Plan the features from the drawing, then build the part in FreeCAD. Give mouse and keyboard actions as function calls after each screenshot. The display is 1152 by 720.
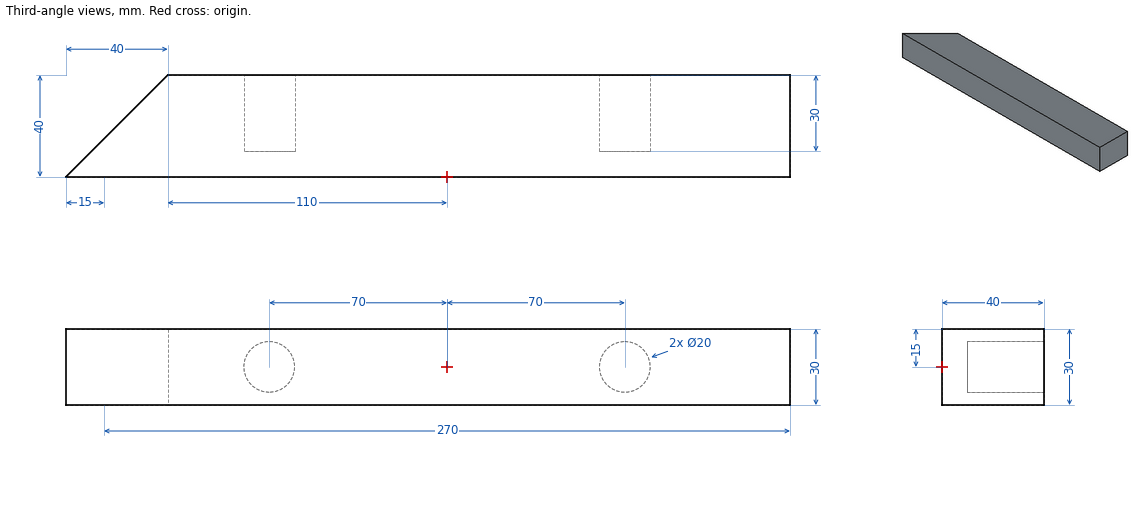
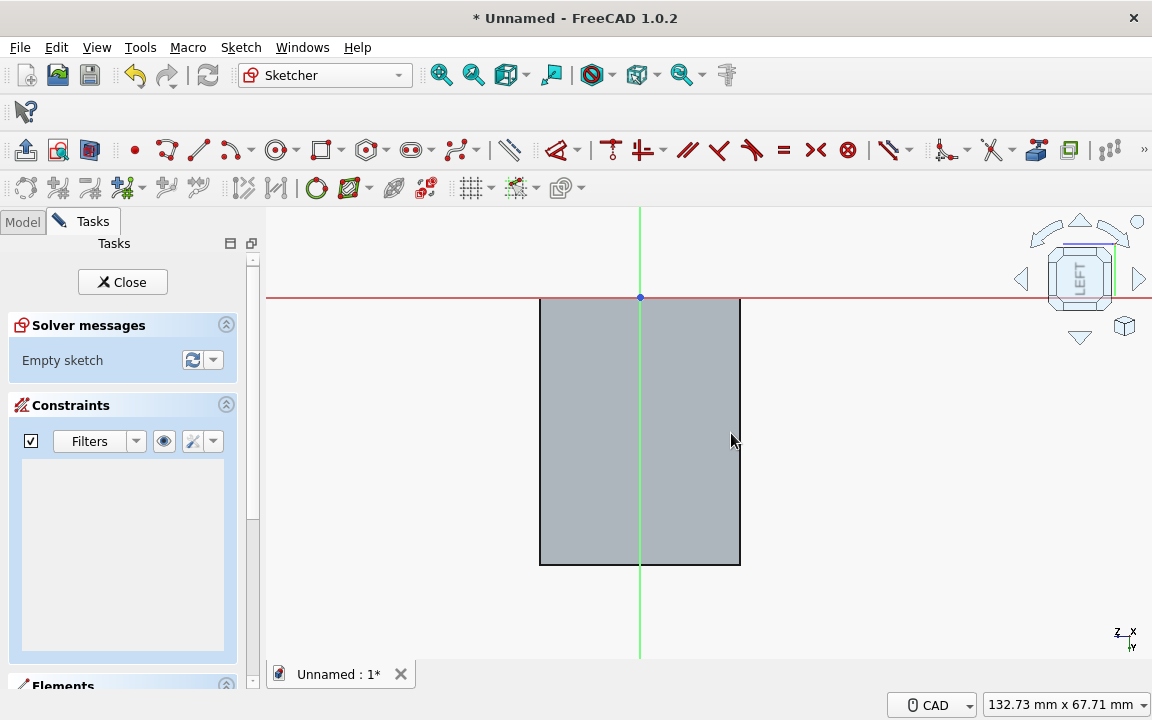
key(g)
key(r)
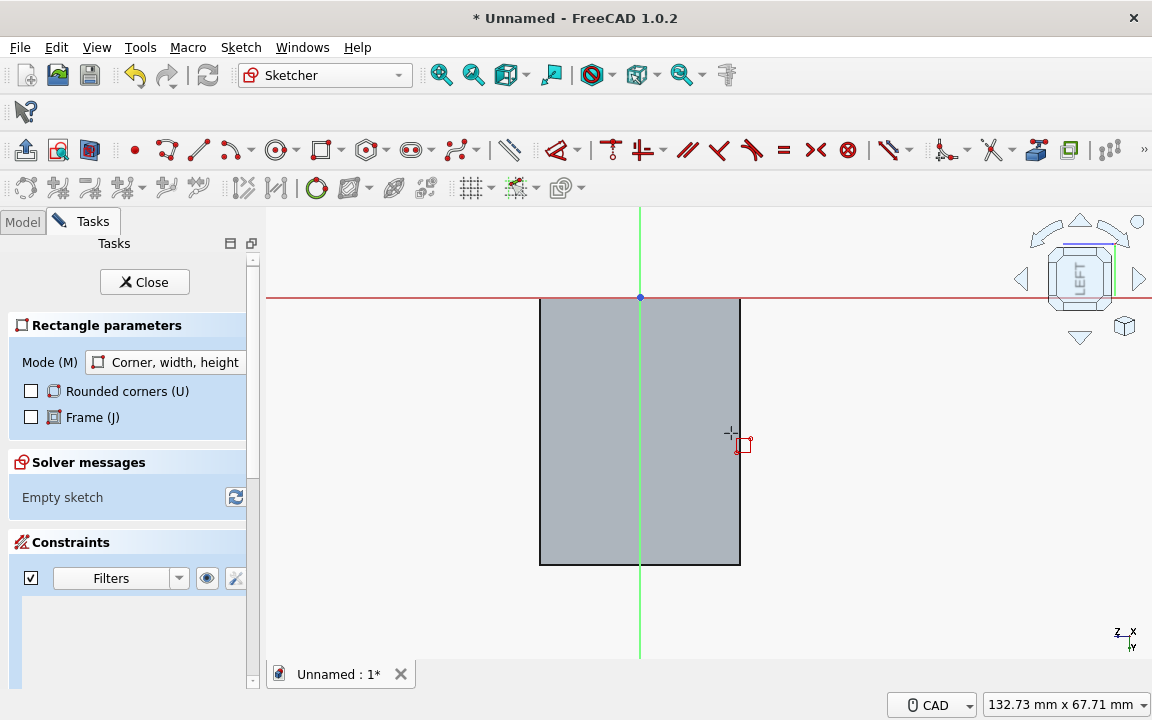
click(540, 298)
move(740, 565)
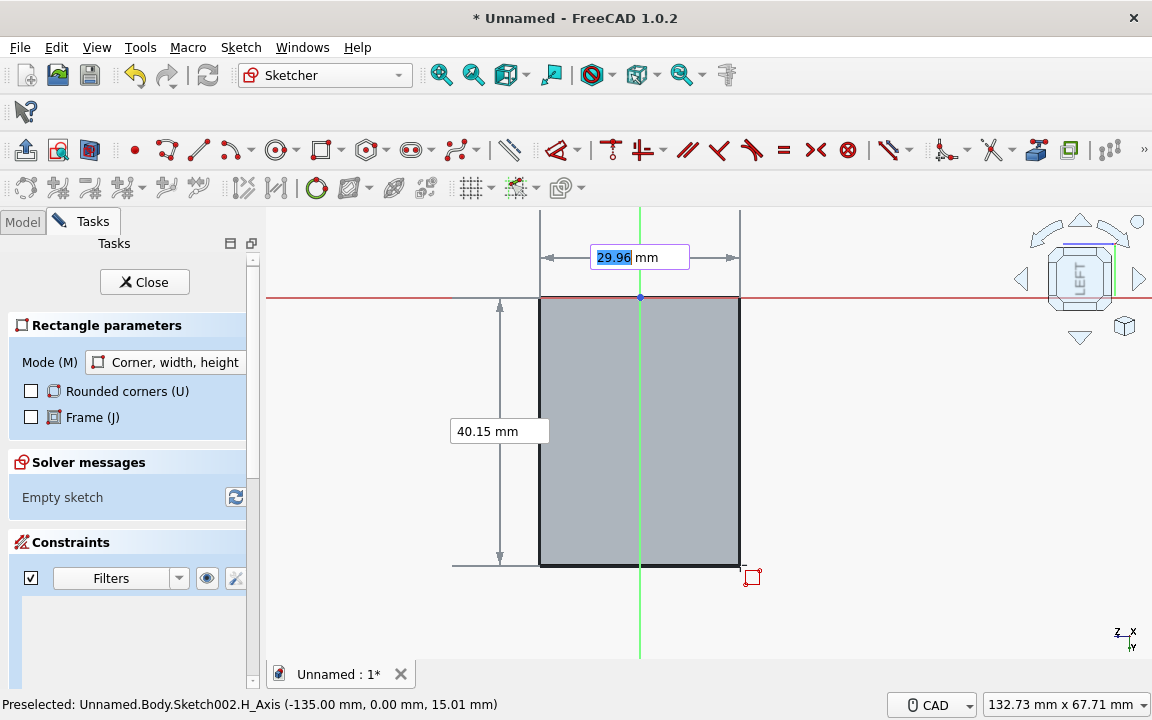
text(30)
key(Tab)
text(40)
key(Return)
key(Escape)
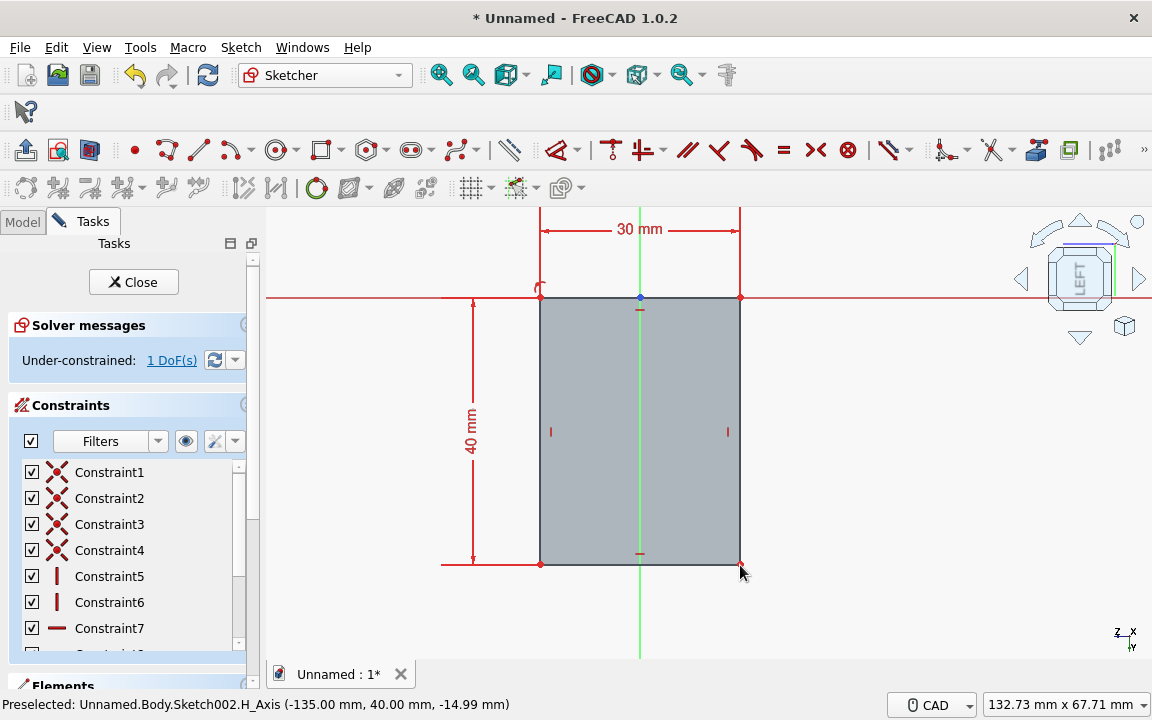
key(d)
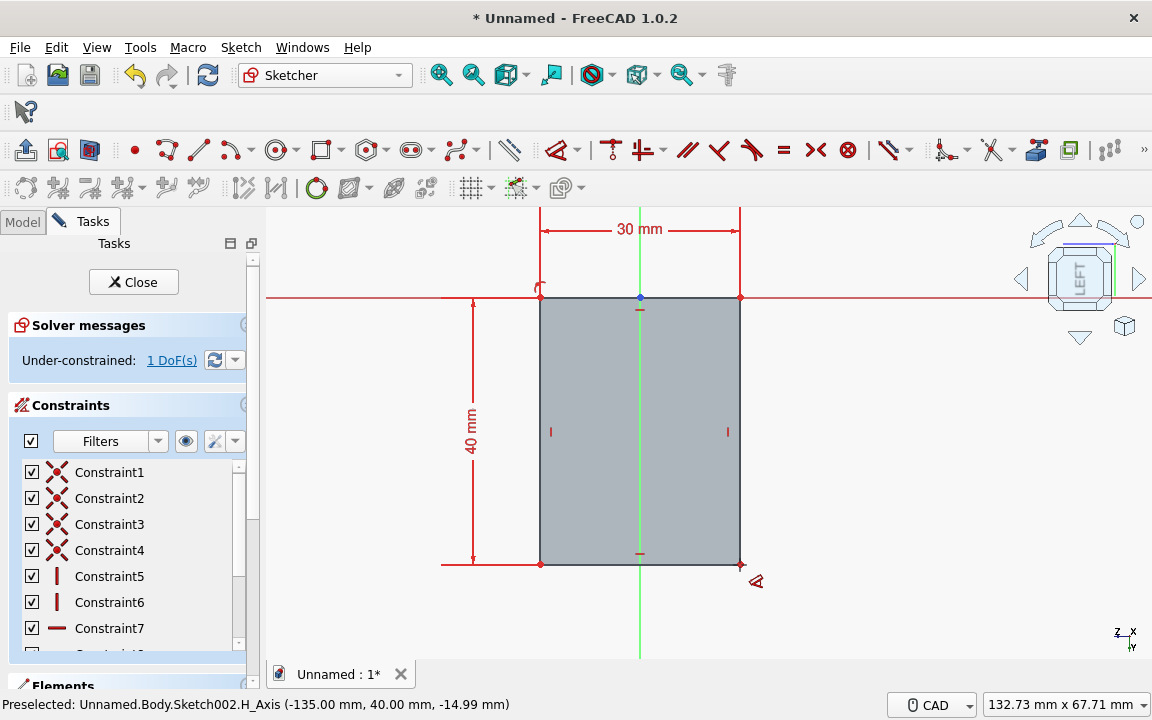
click(540, 298)
click(590, 264)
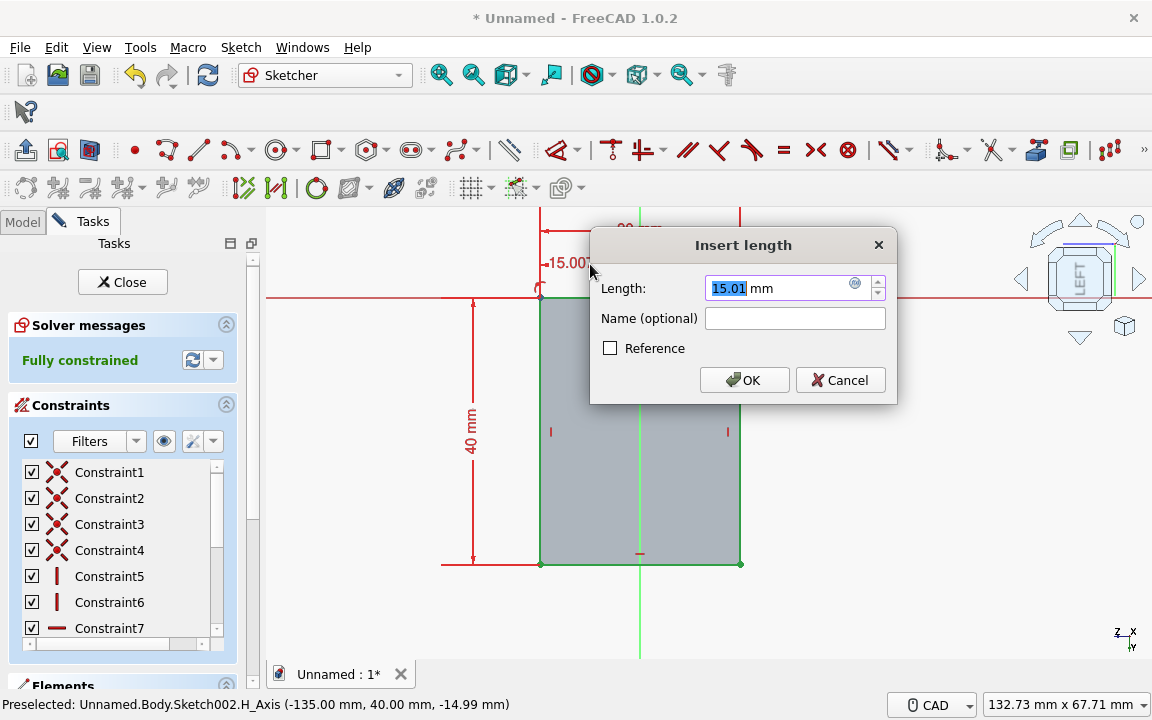
text(15)
key(Return)
key(Escape)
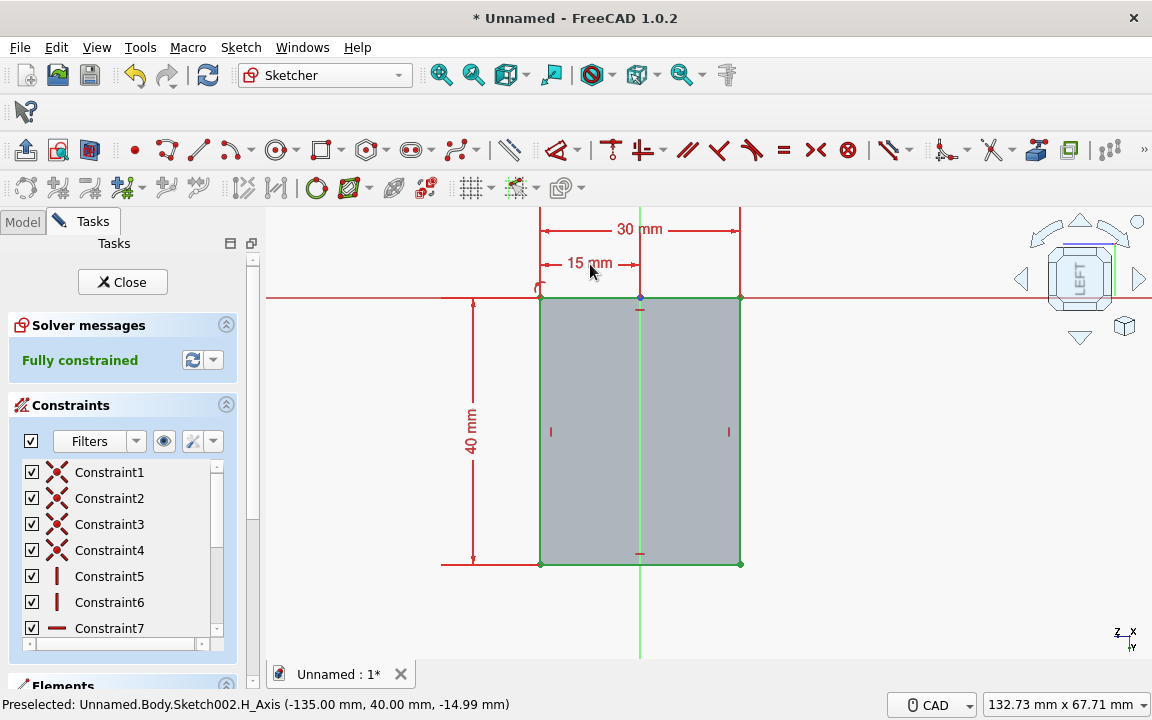
click(123, 282)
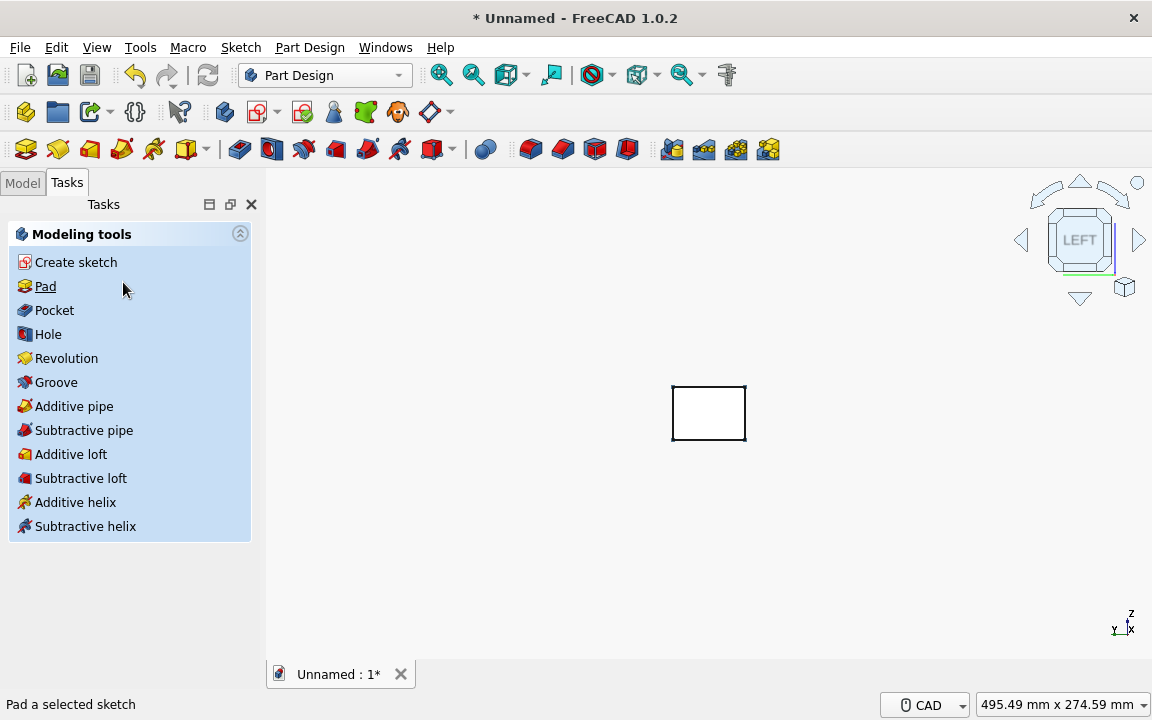
click(26, 150)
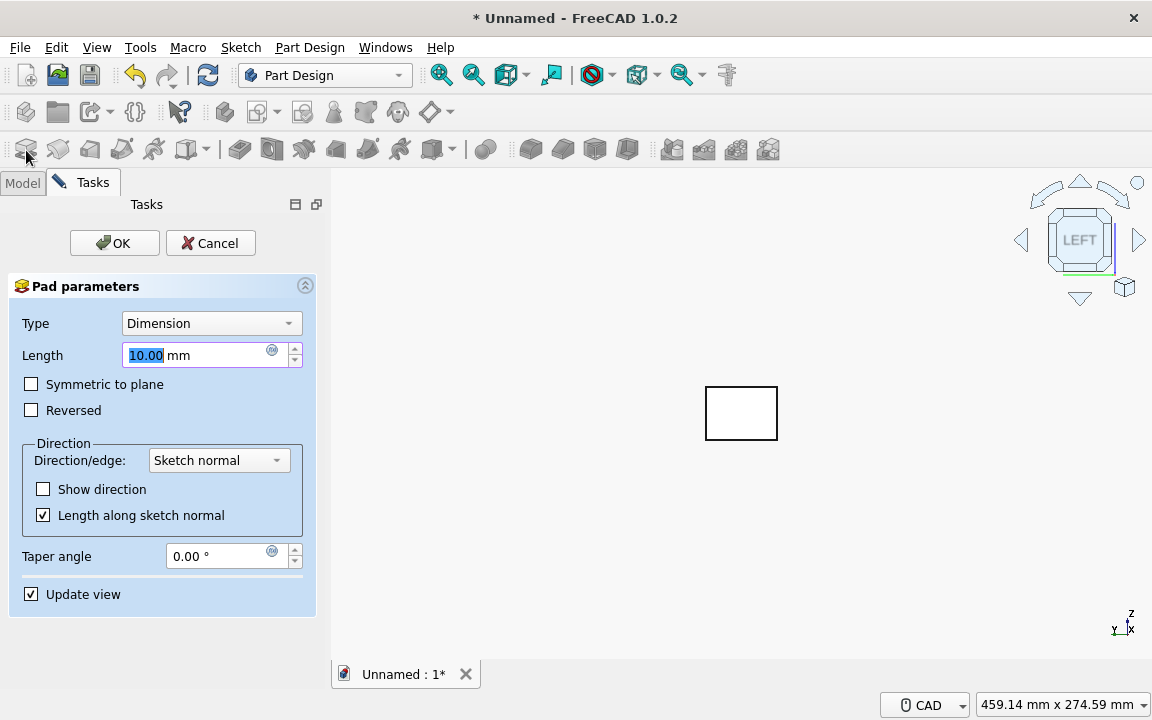
text(15)
key(Tab)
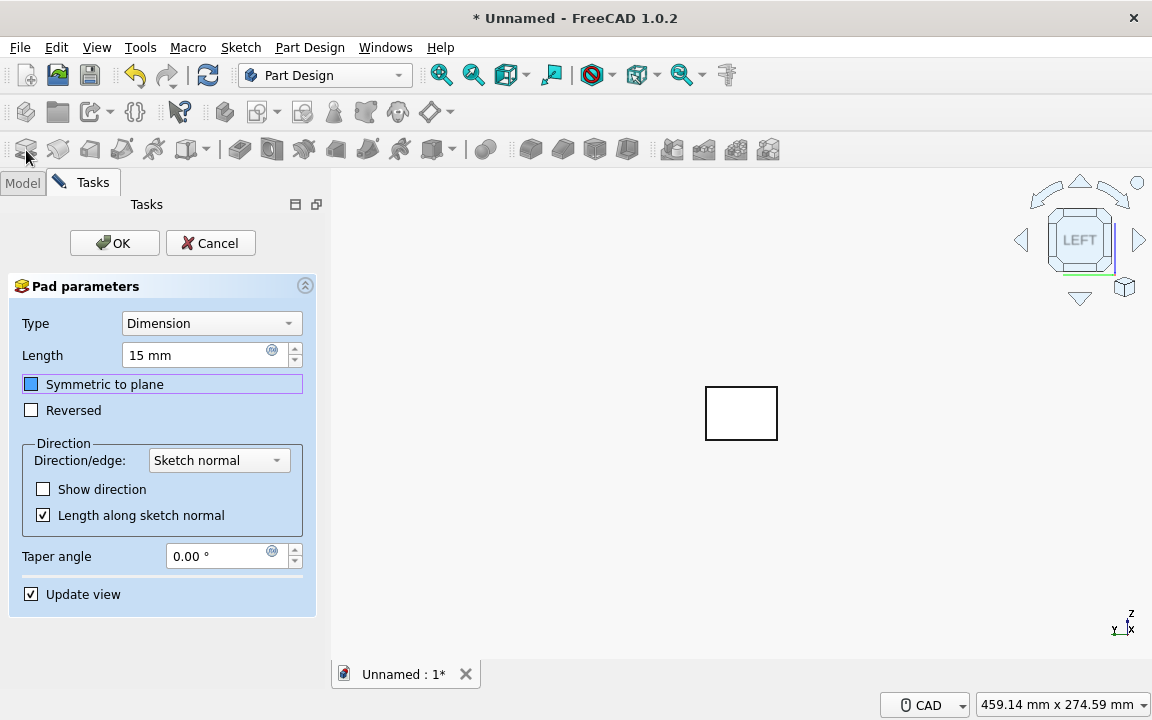
click(115, 243)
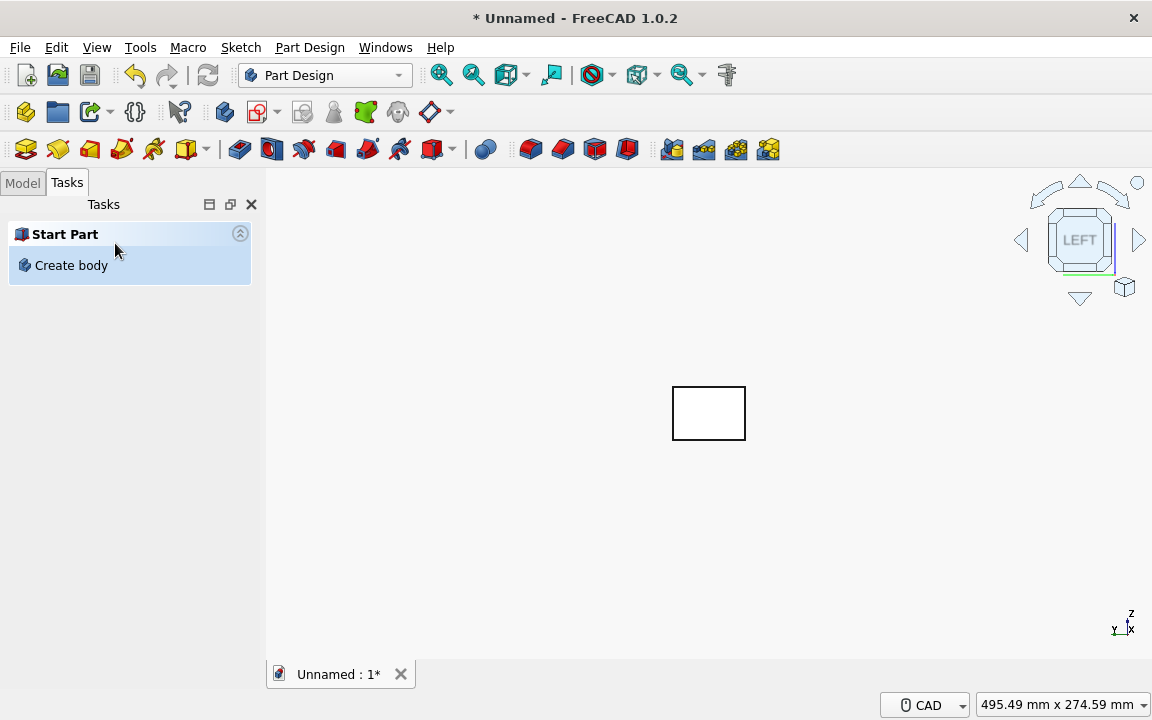
click(442, 76)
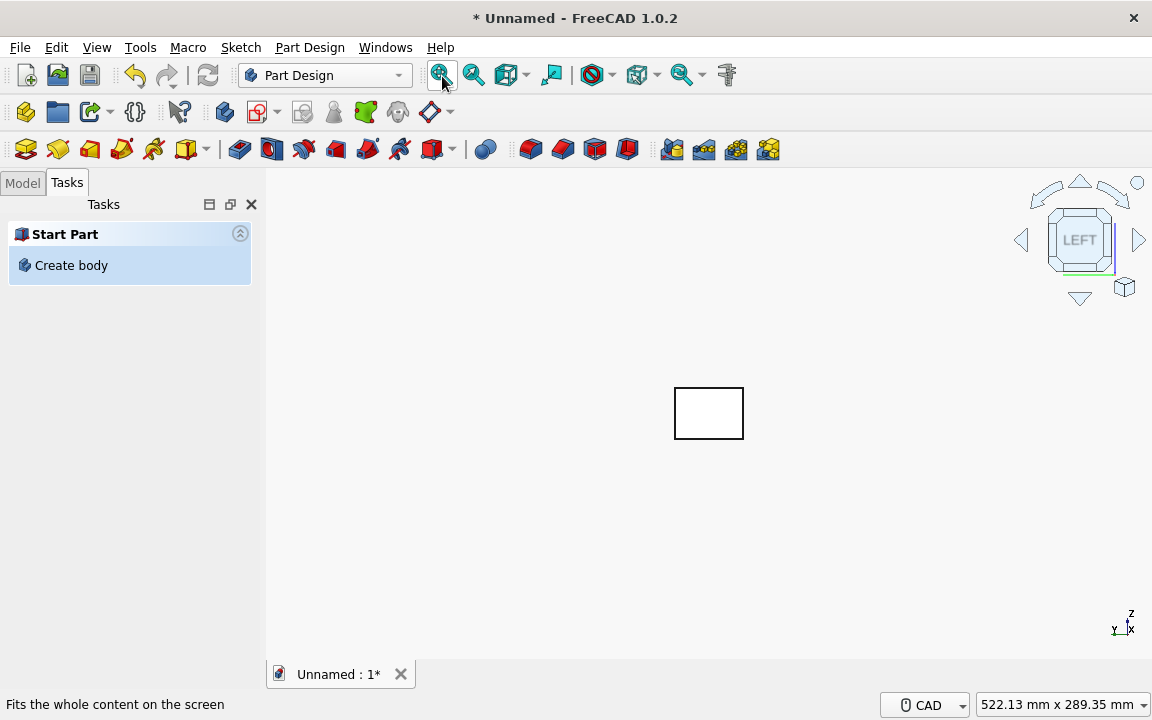
key(0)